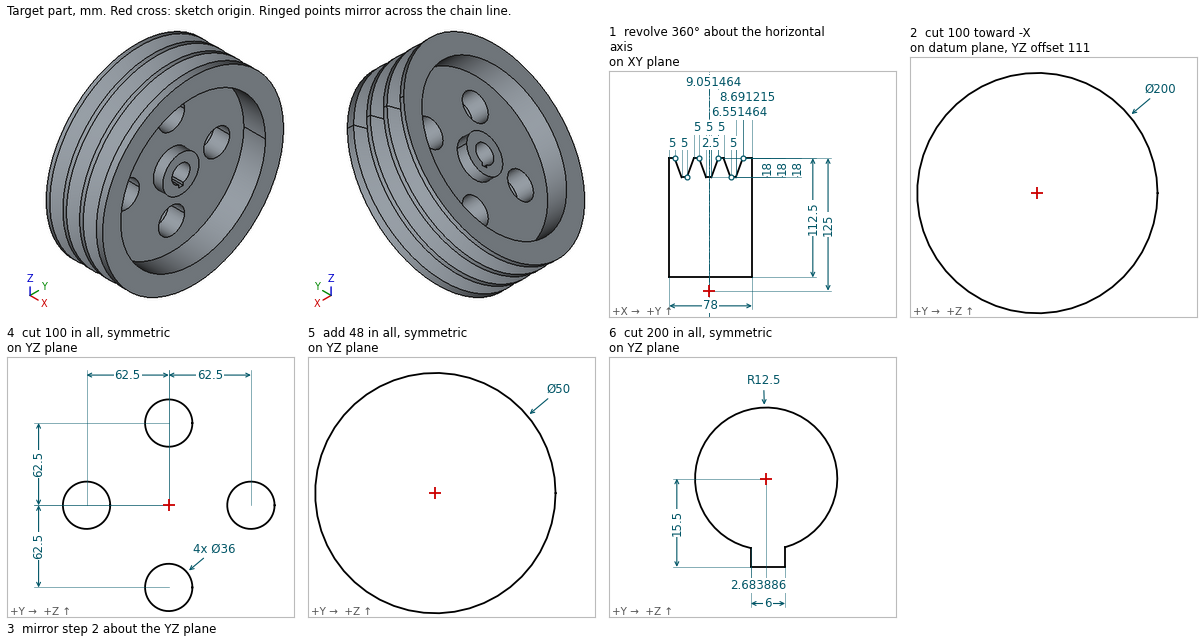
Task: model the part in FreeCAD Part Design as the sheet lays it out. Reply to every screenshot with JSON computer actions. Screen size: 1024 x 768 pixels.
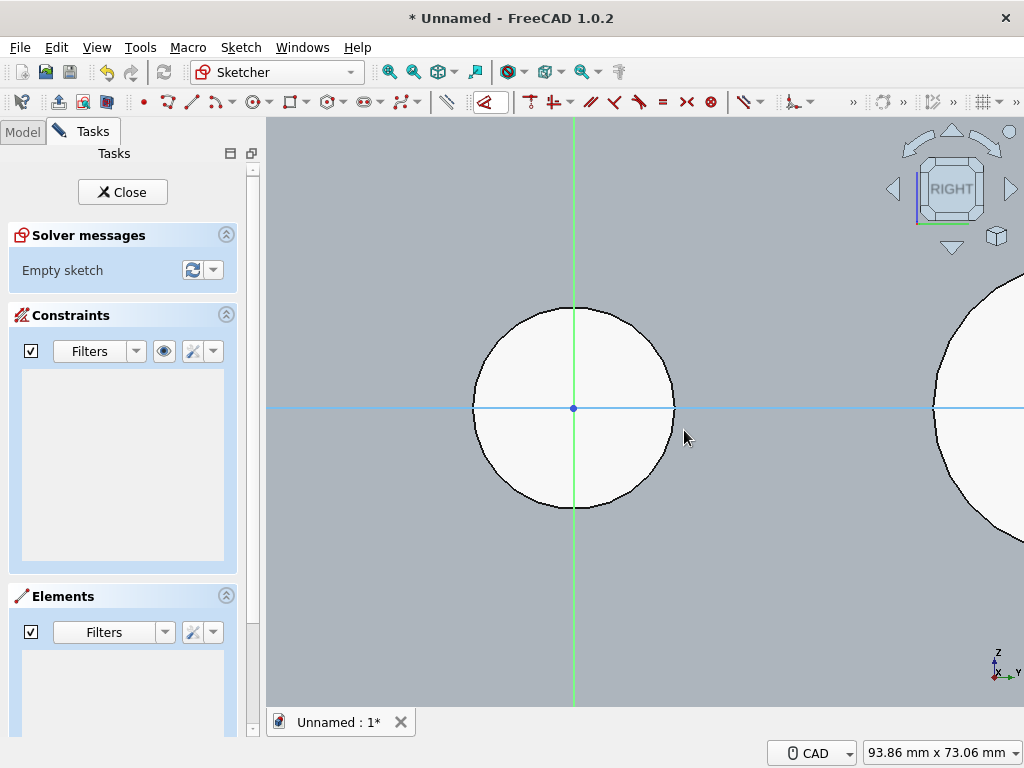
{"action": "left_click", "coordinate": [254, 102]}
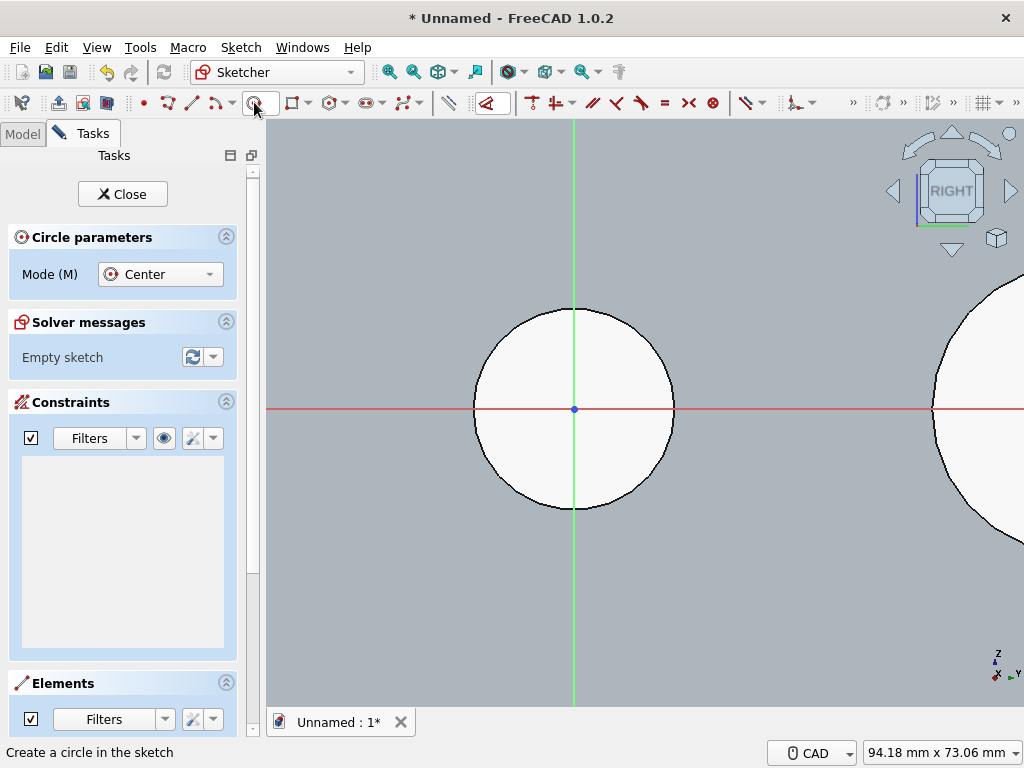
{"action": "left_click", "coordinate": [574, 409]}
{"action": "left_click", "coordinate": [716, 267]}
{"action": "key", "text": "Escape"}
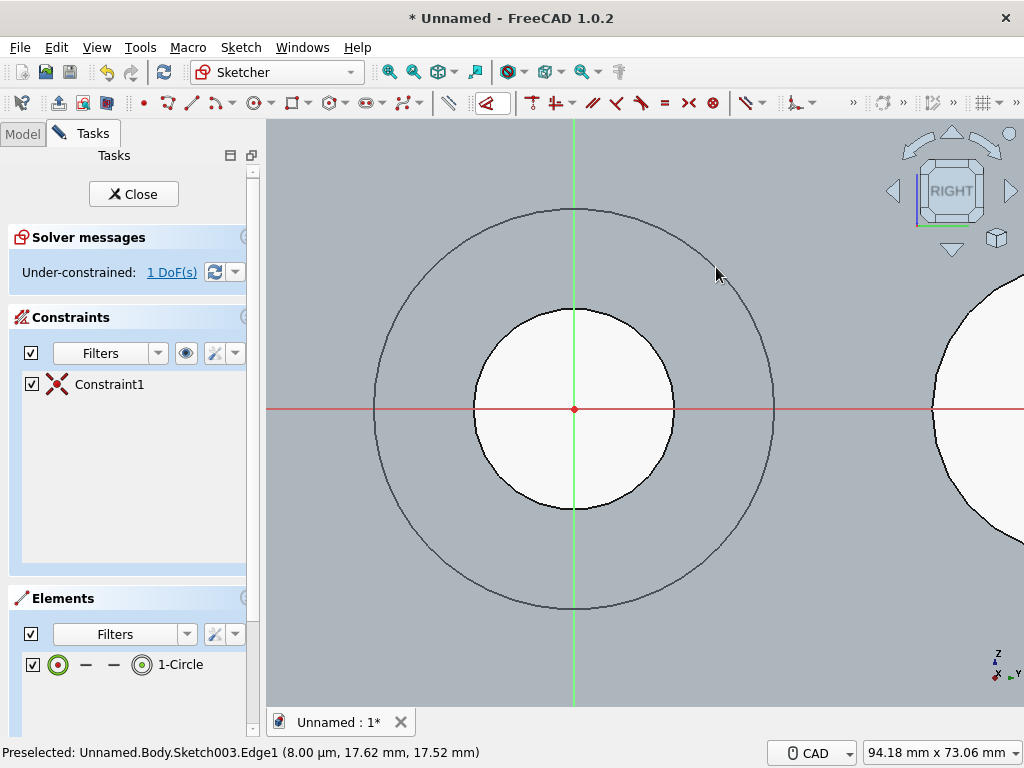
{"action": "left_click", "coordinate": [715, 267]}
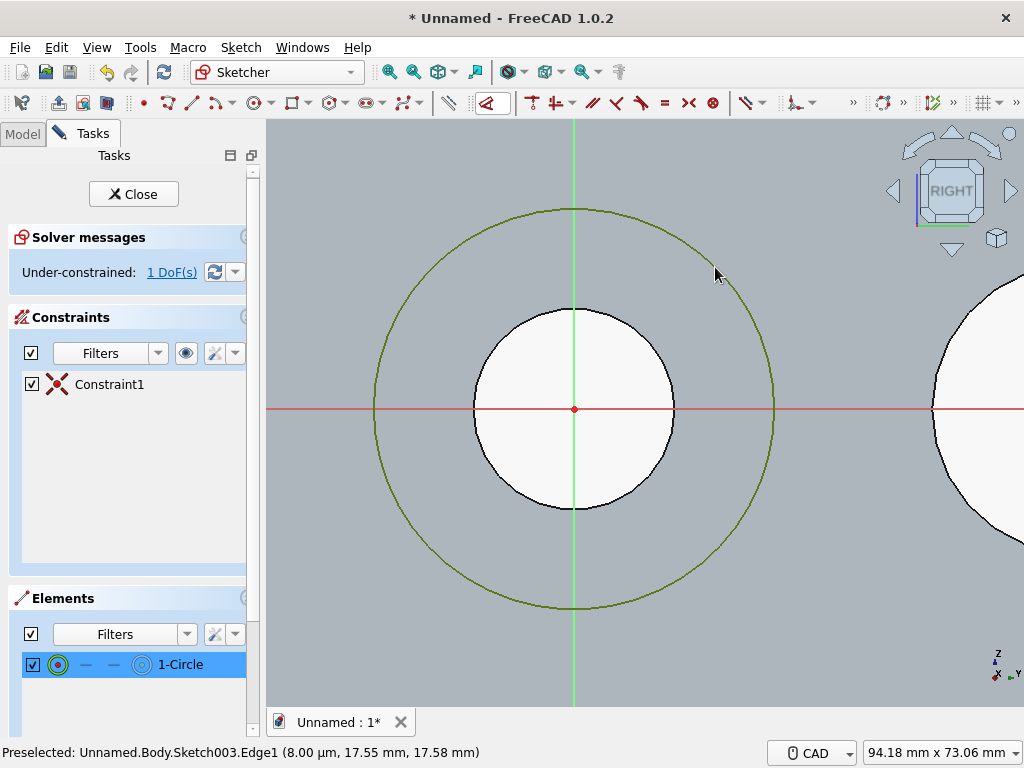
{"action": "key", "text": "k o"}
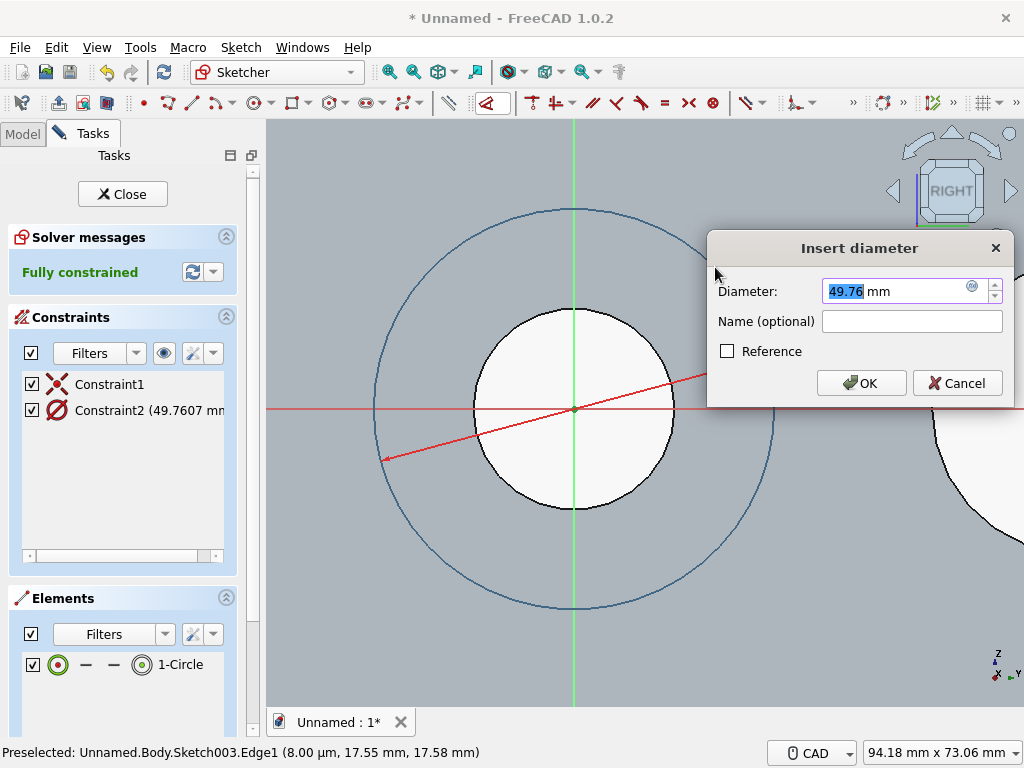
{"action": "type", "text": "50"}
{"action": "key", "text": "Return"}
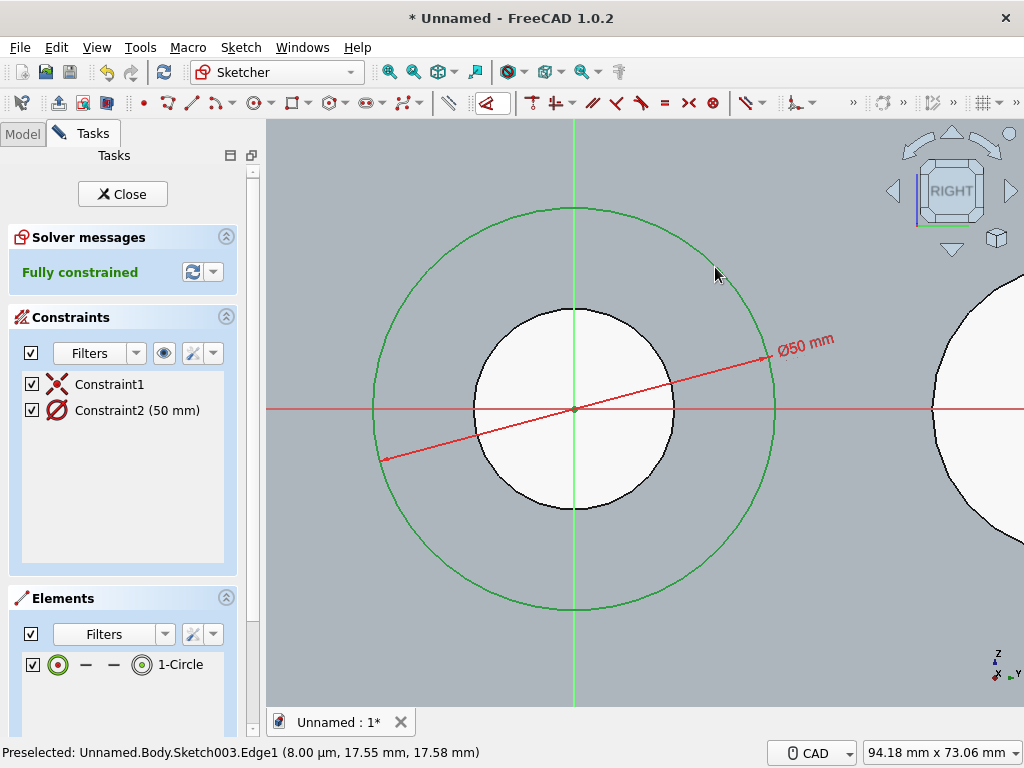
{"action": "left_click", "coordinate": [123, 194]}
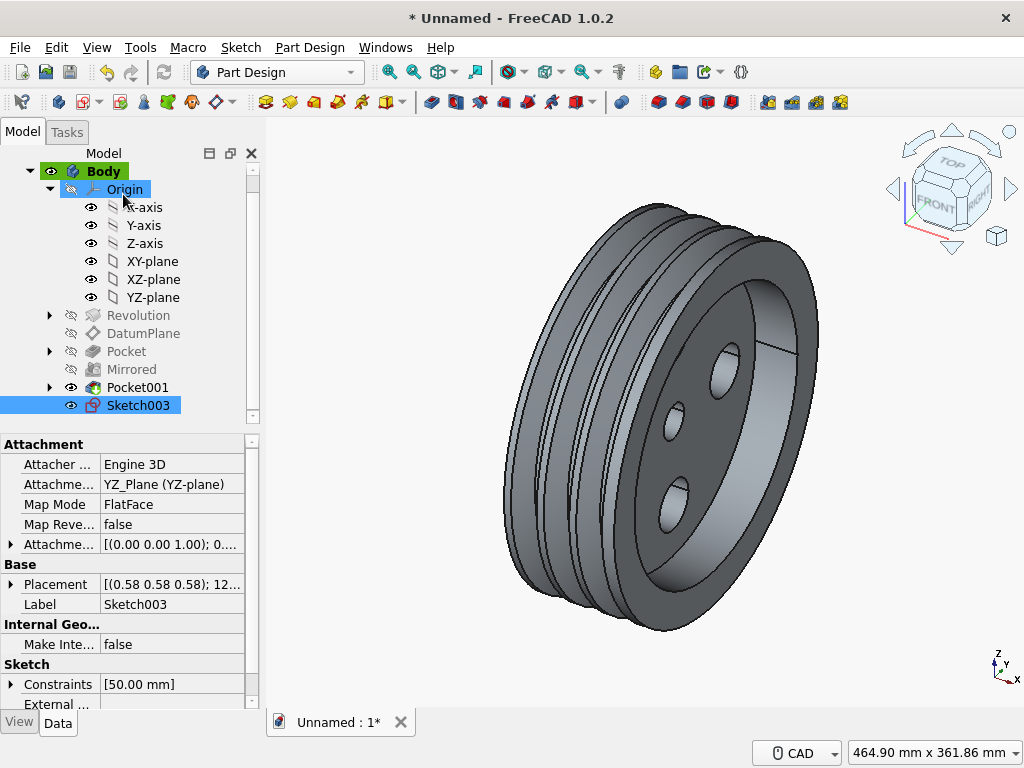
{"action": "left_click", "coordinate": [266, 102]}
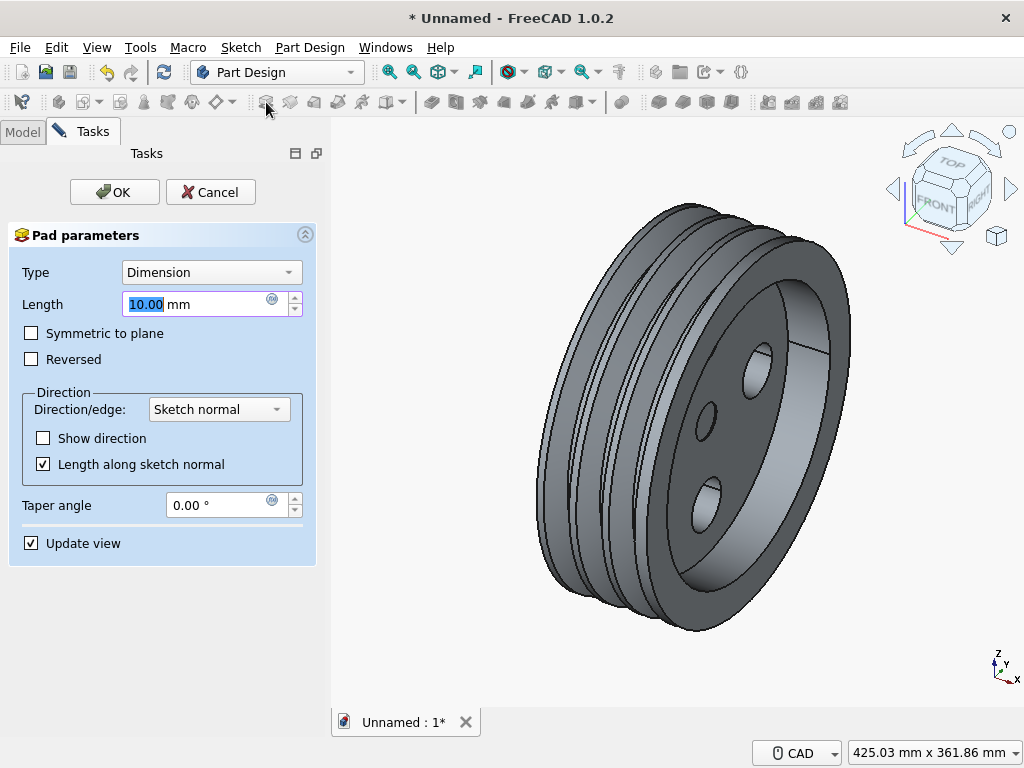
{"action": "type", "text": "48"}
{"action": "key", "text": "Tab"}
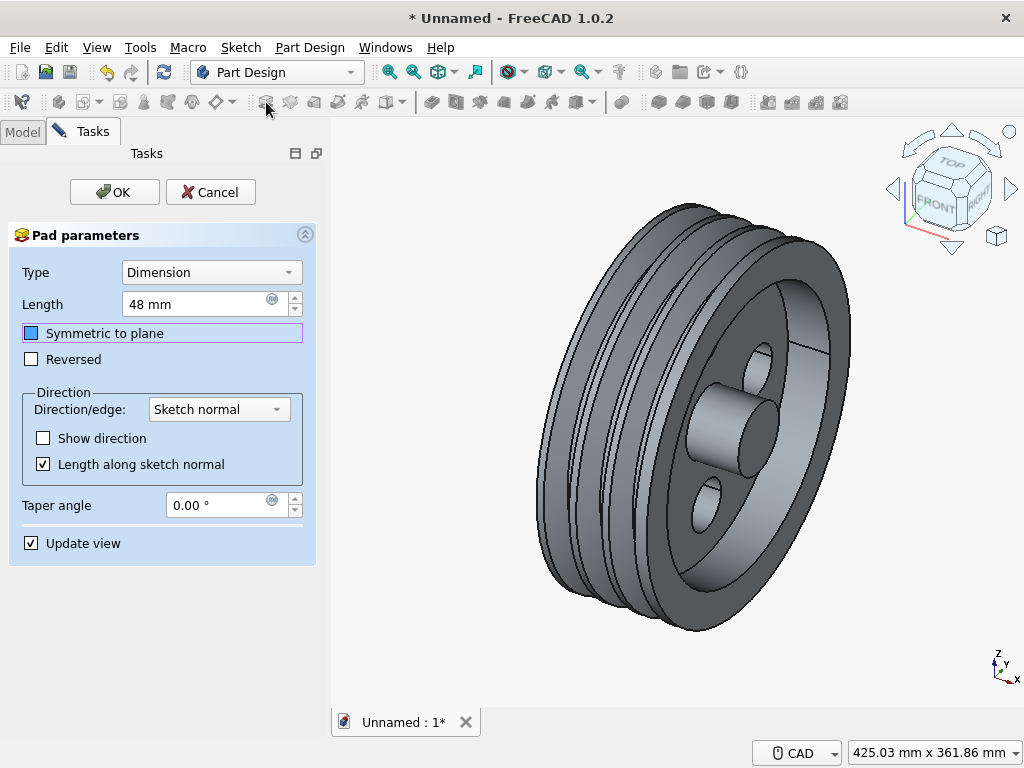
{"action": "left_click", "coordinate": [30, 333]}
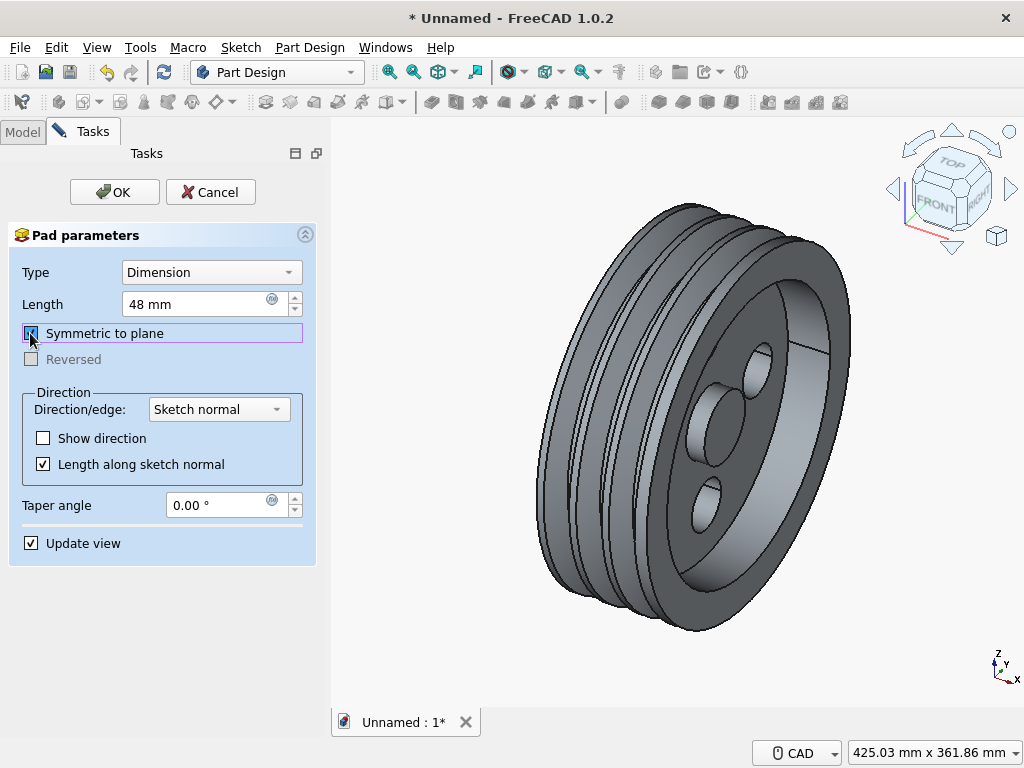
{"action": "left_click", "coordinate": [115, 192]}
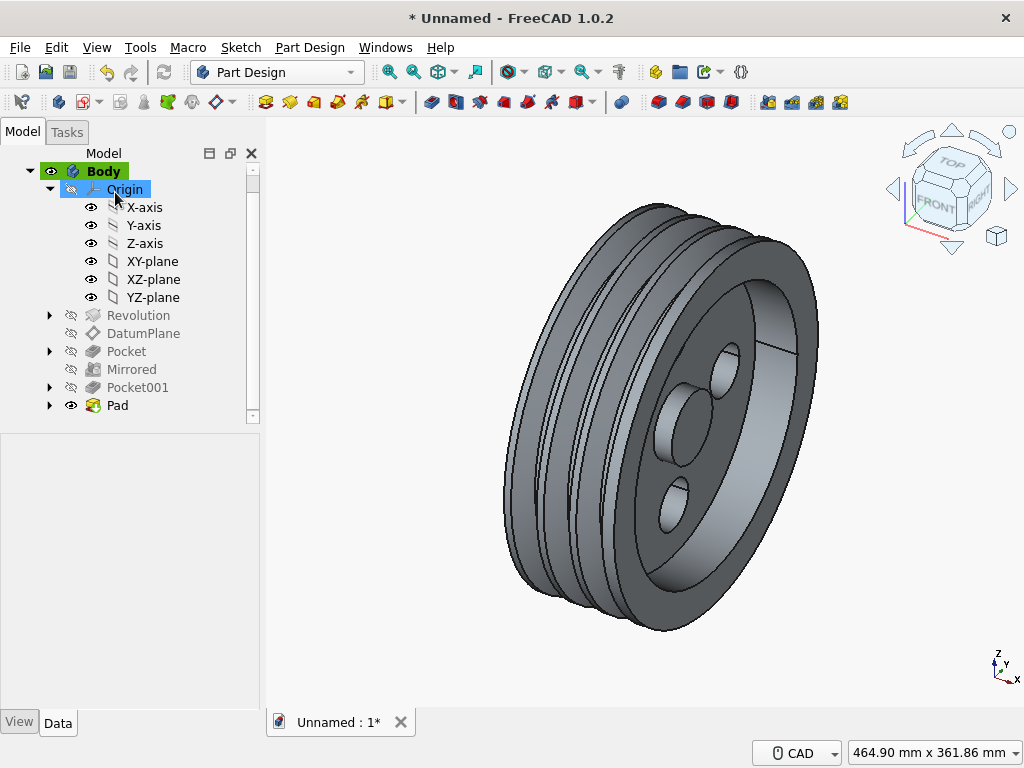
{"action": "left_click", "coordinate": [84, 102]}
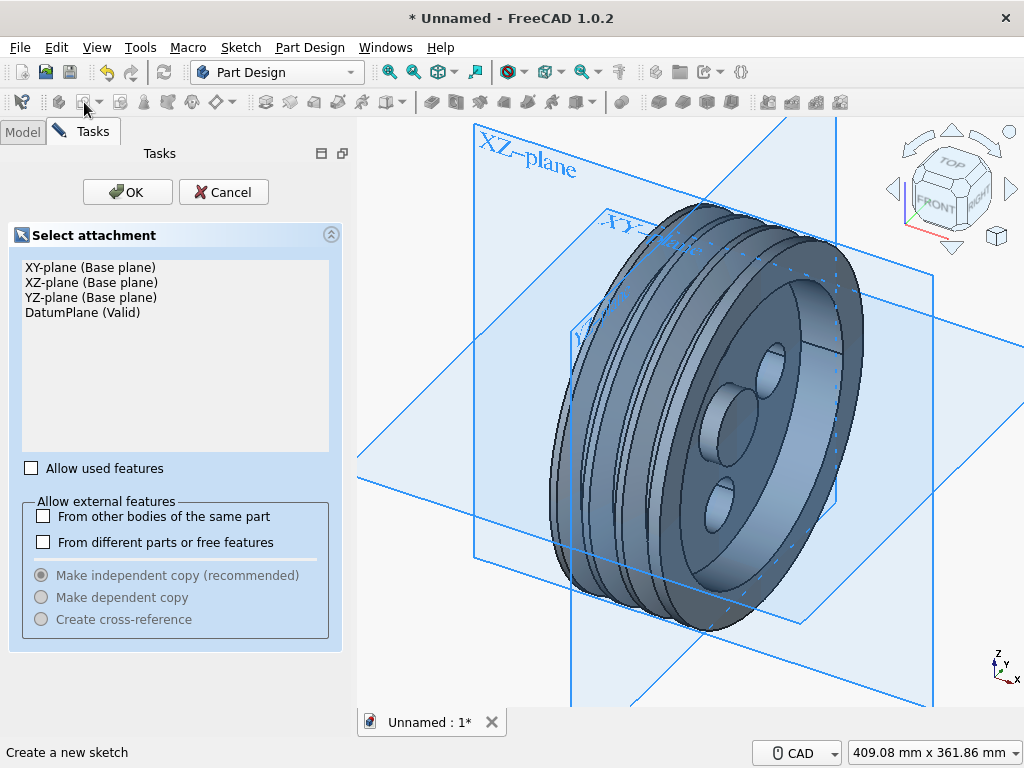
{"action": "left_click", "coordinate": [82, 298]}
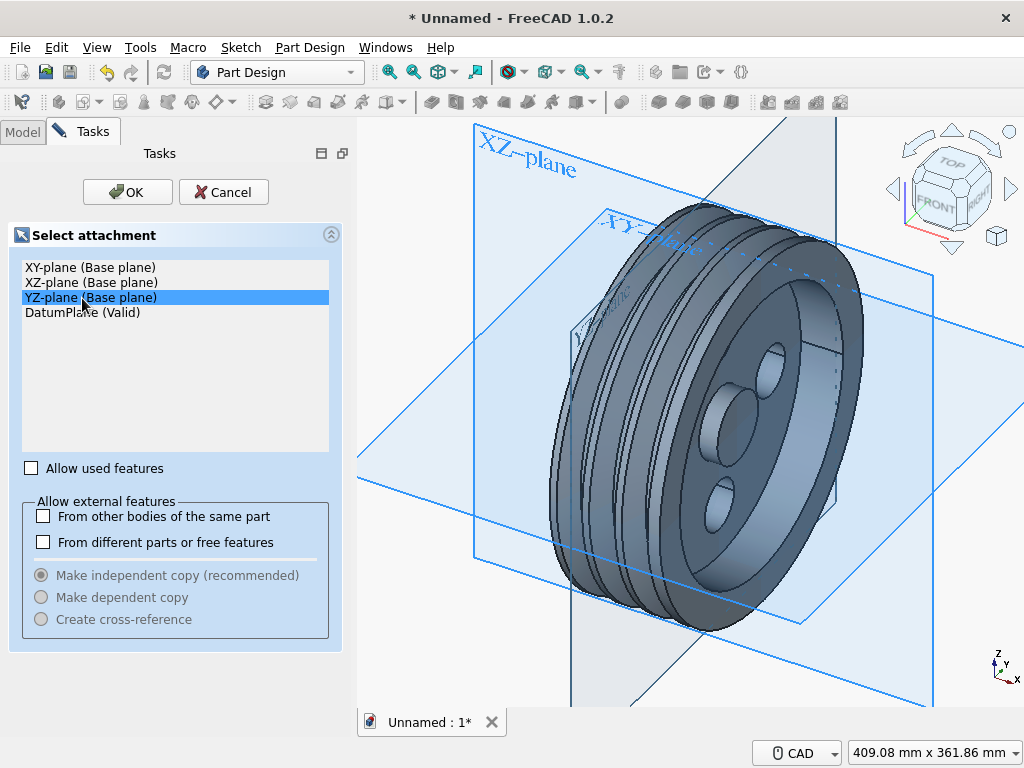
{"action": "left_click", "coordinate": [128, 192]}